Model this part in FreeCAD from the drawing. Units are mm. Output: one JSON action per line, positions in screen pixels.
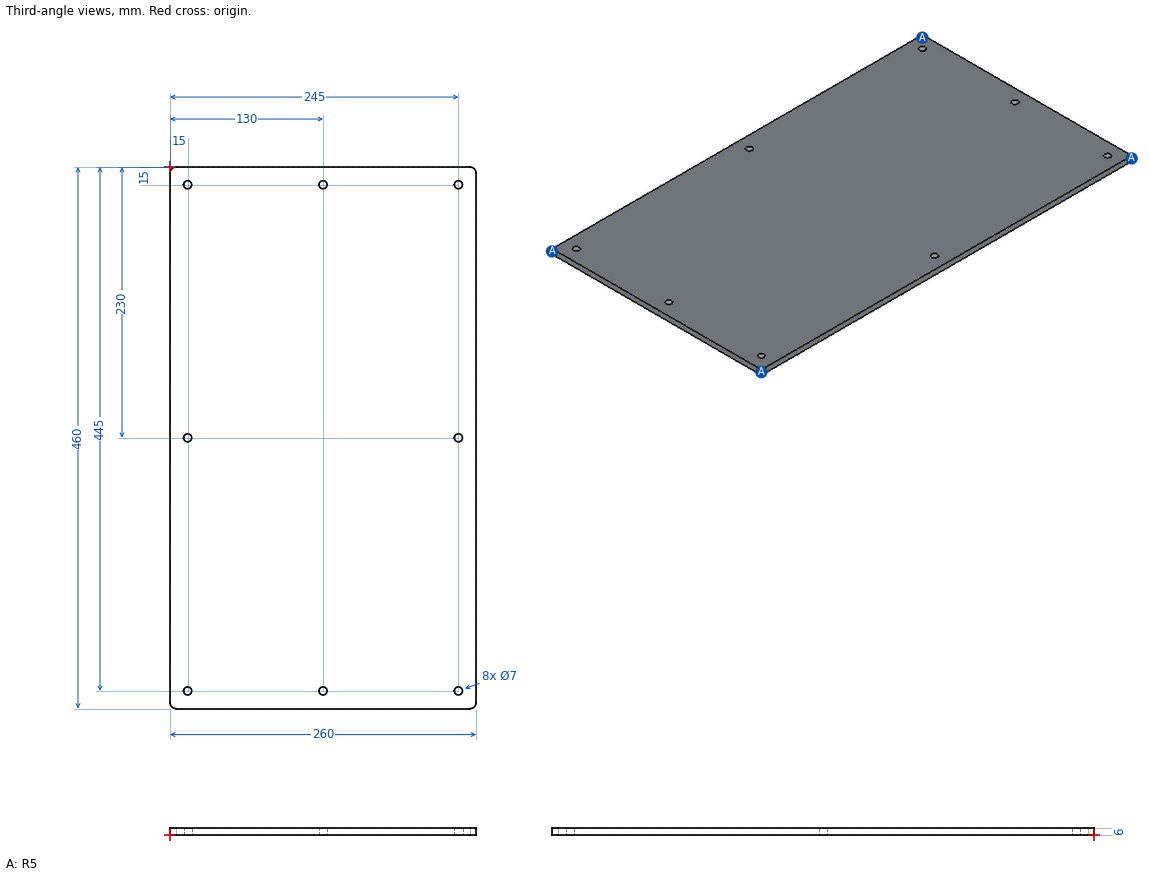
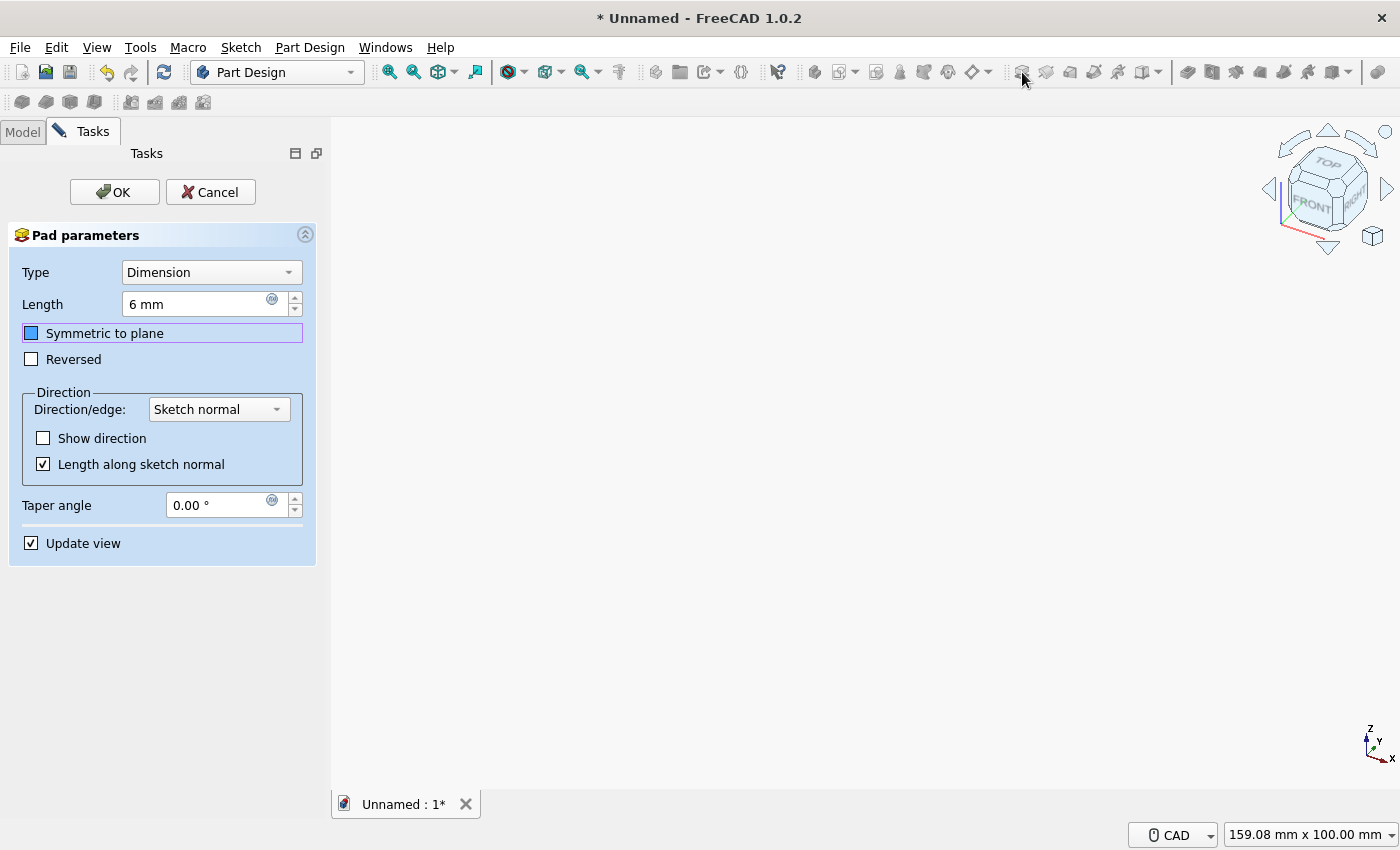
{"action": "left_click", "coordinate": [115, 192]}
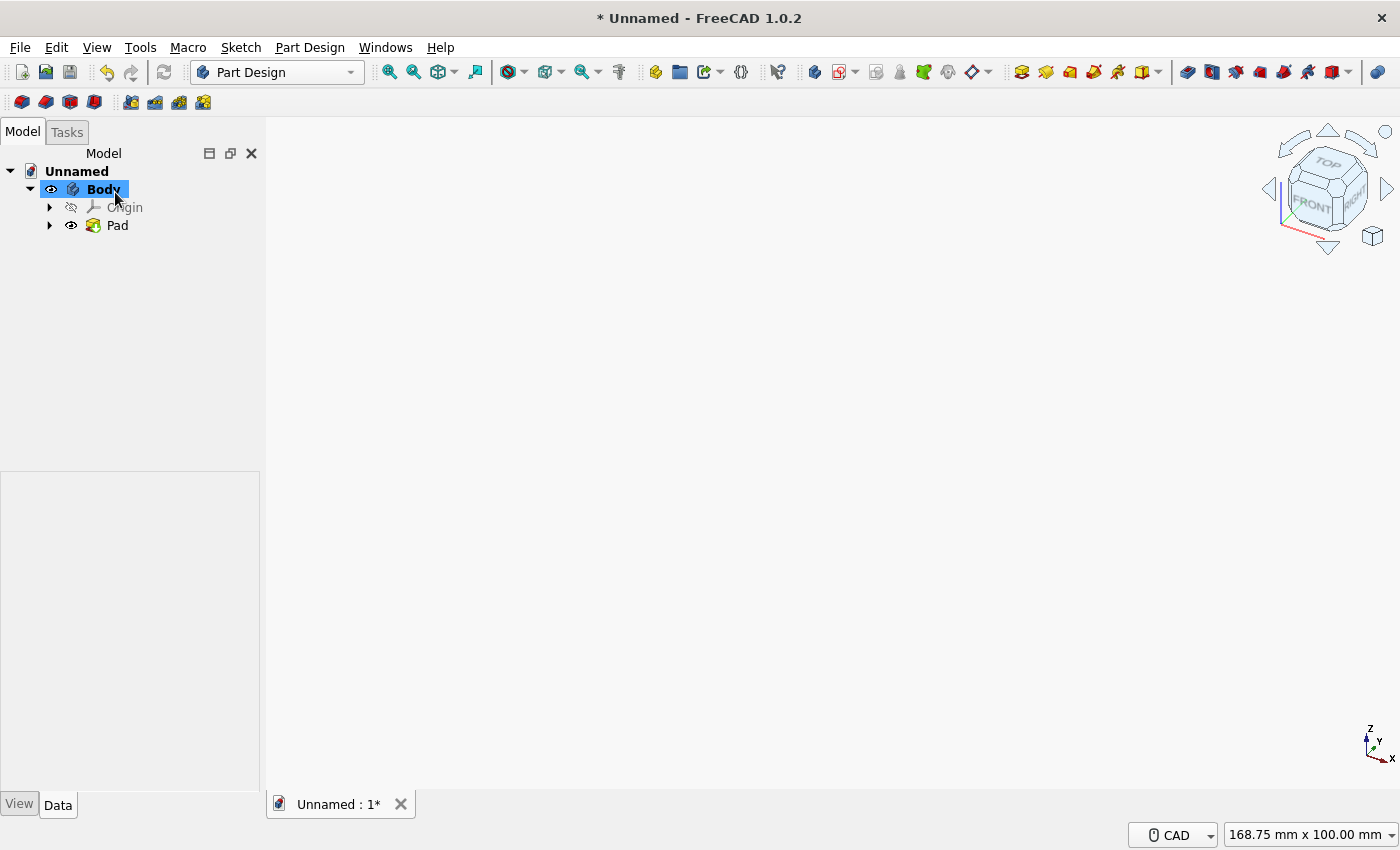
{"action": "key", "text": "v f"}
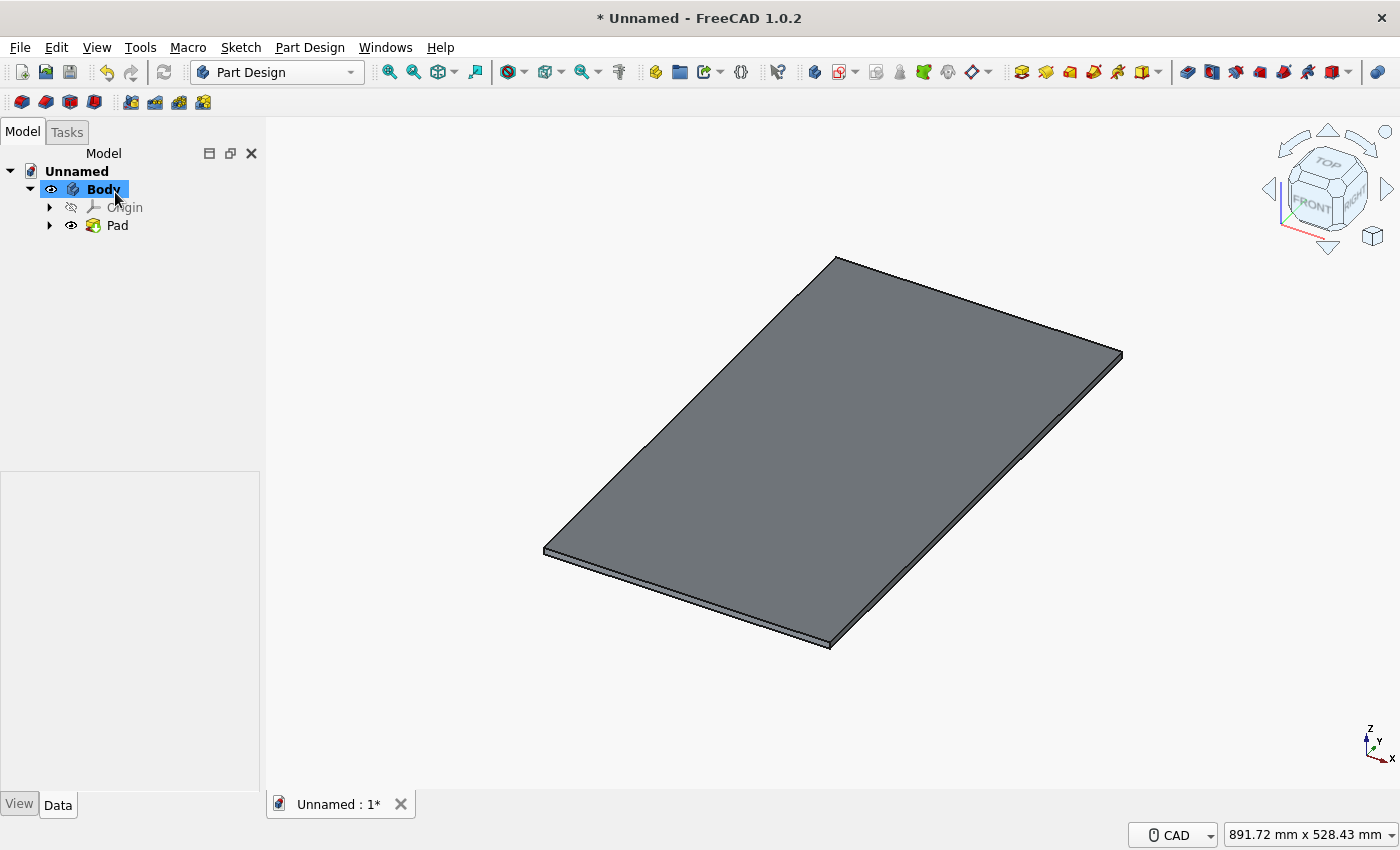
{"action": "scroll", "coordinate": [836, 259], "scroll_direction": "up", "scroll_amount": 9}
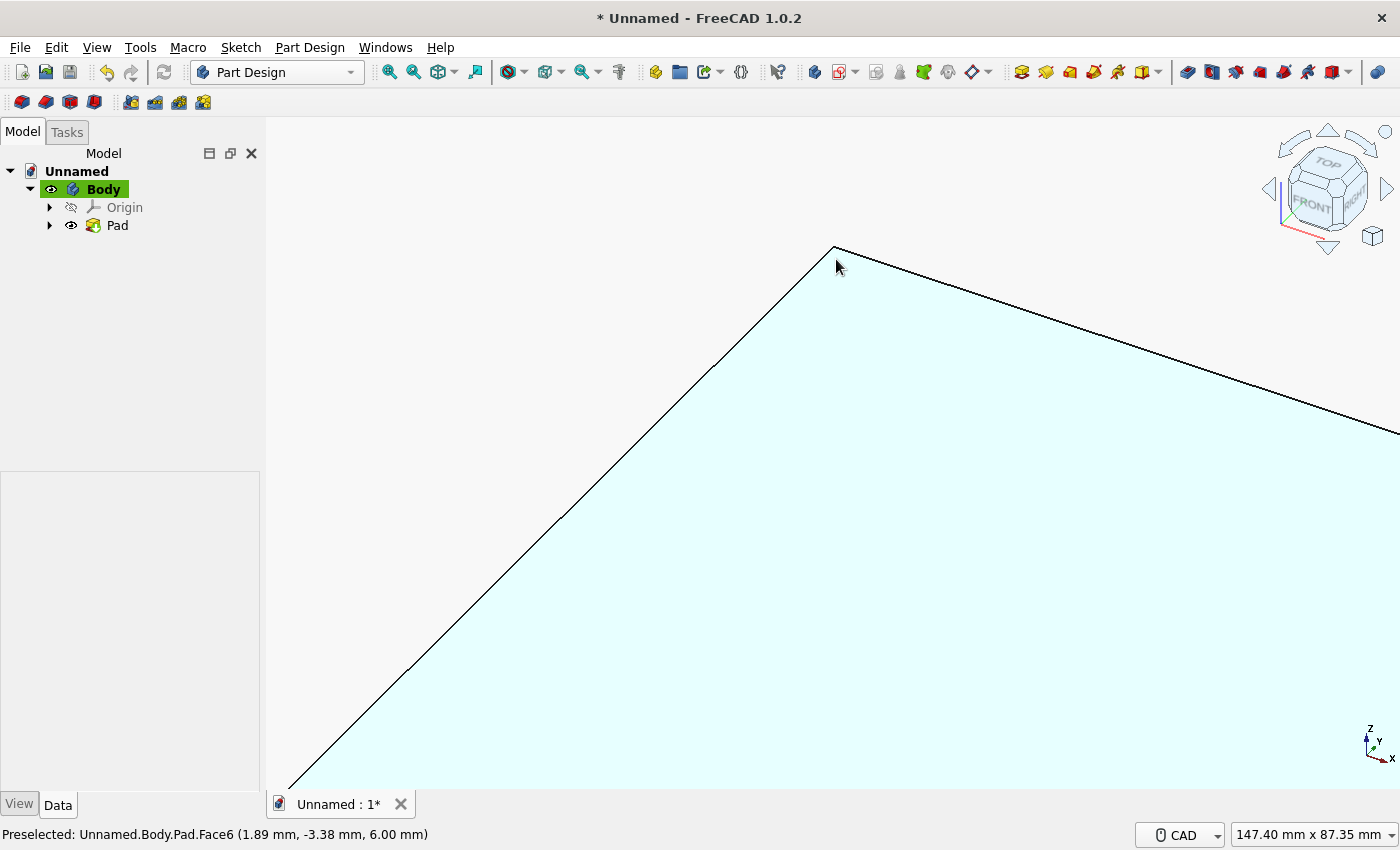
{"action": "key", "text": "v f"}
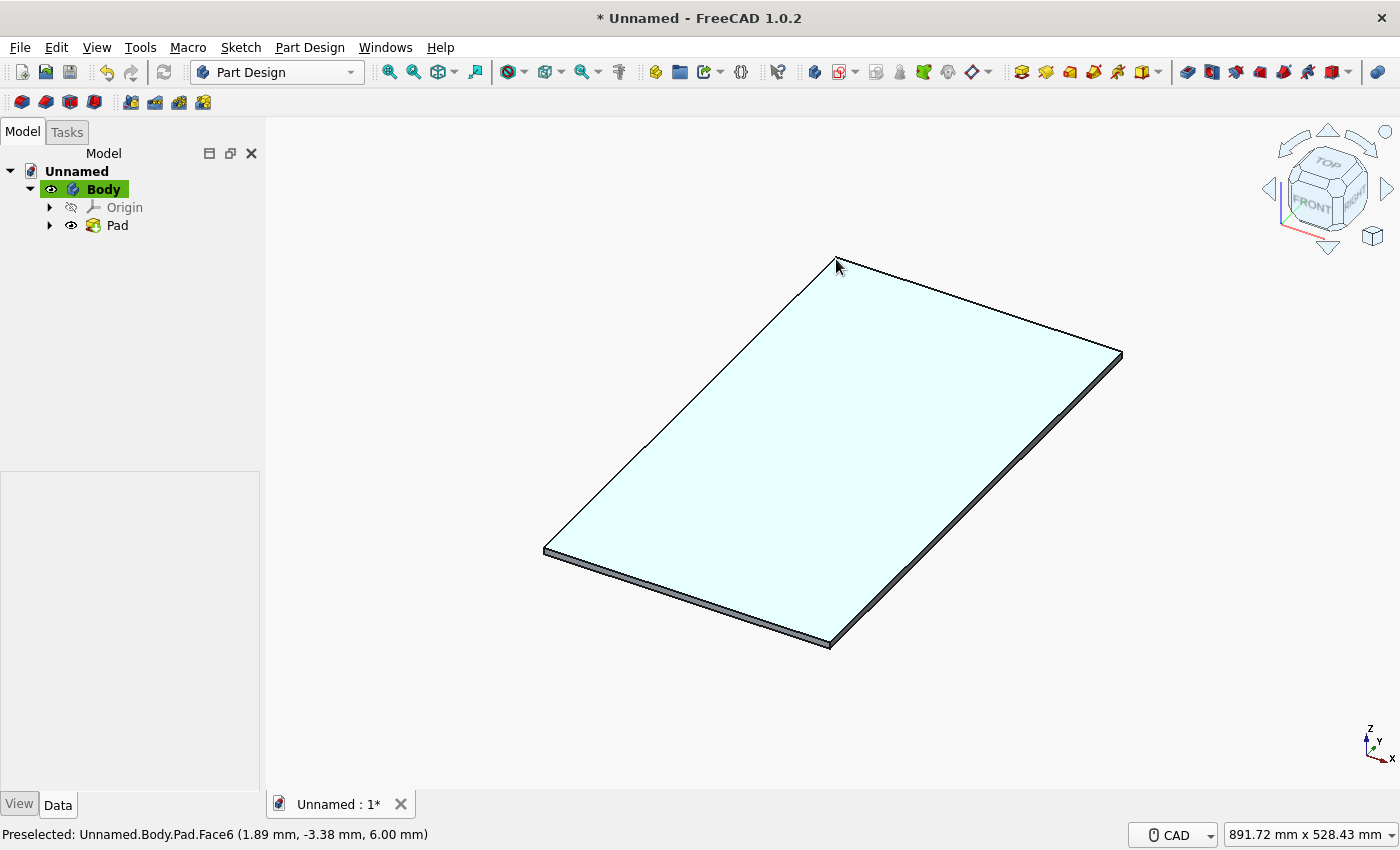
{"action": "key", "text": "0"}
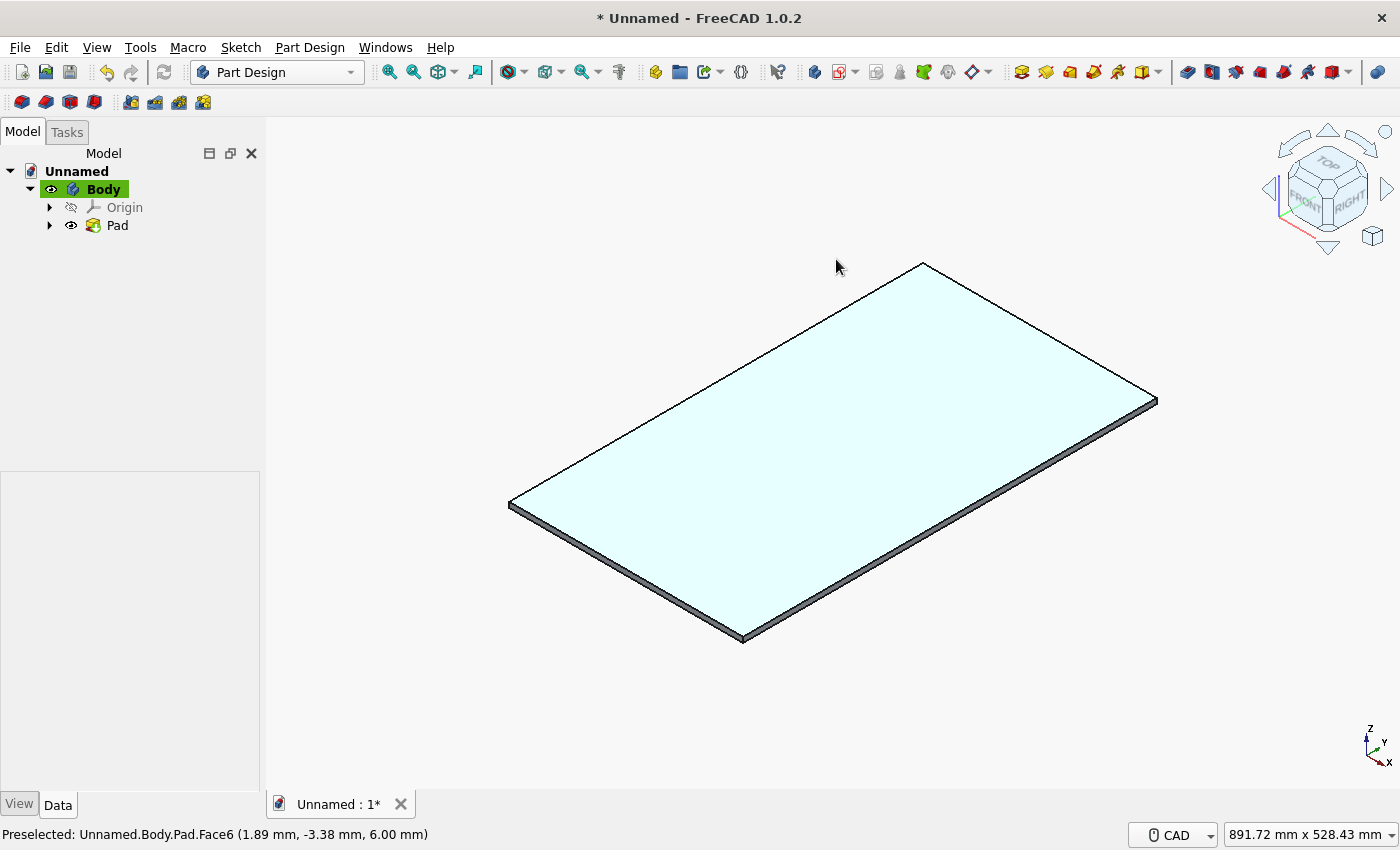
{"action": "scroll", "coordinate": [923, 265], "scroll_direction": "up", "scroll_amount": 9}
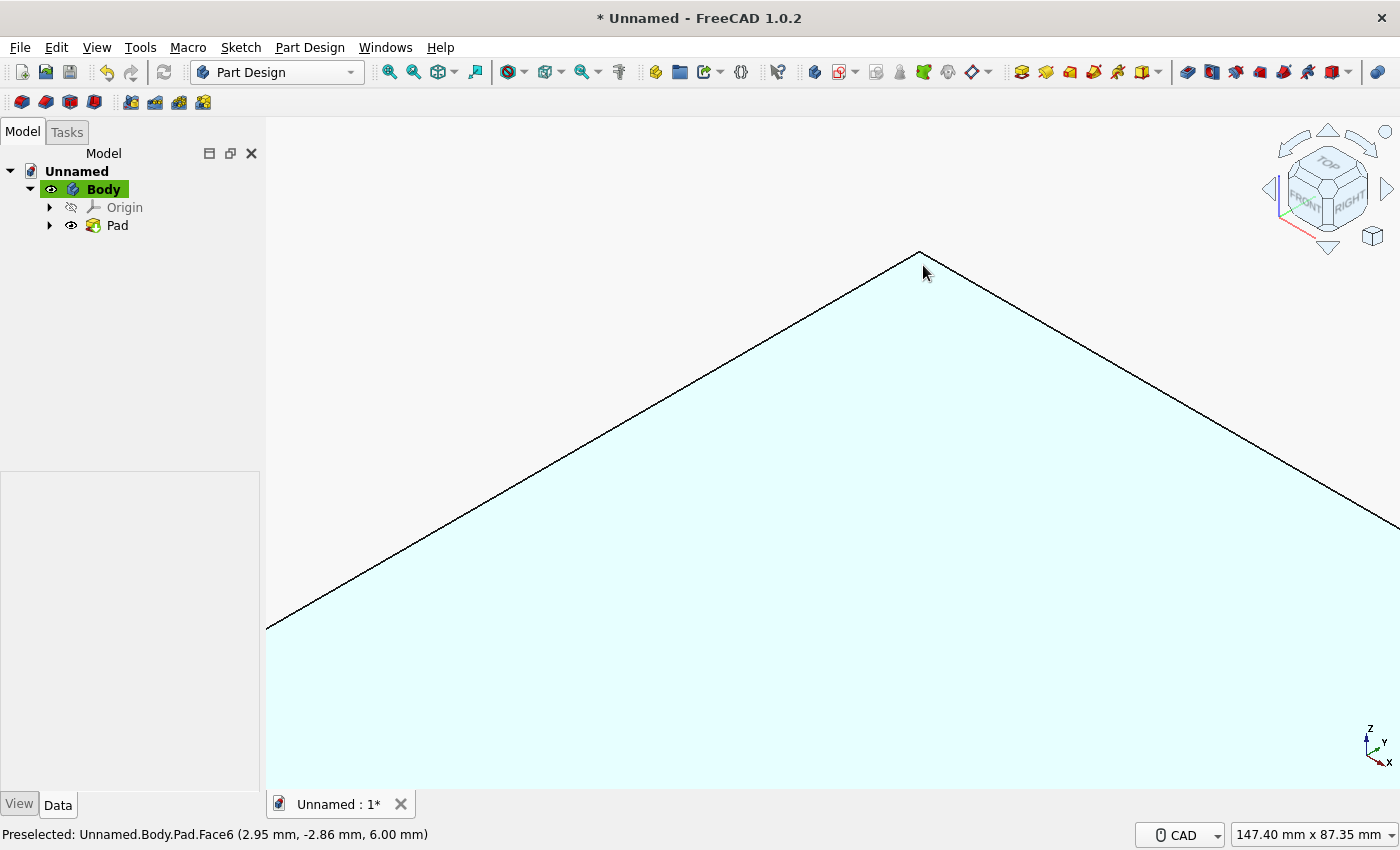
{"action": "key", "text": "v f"}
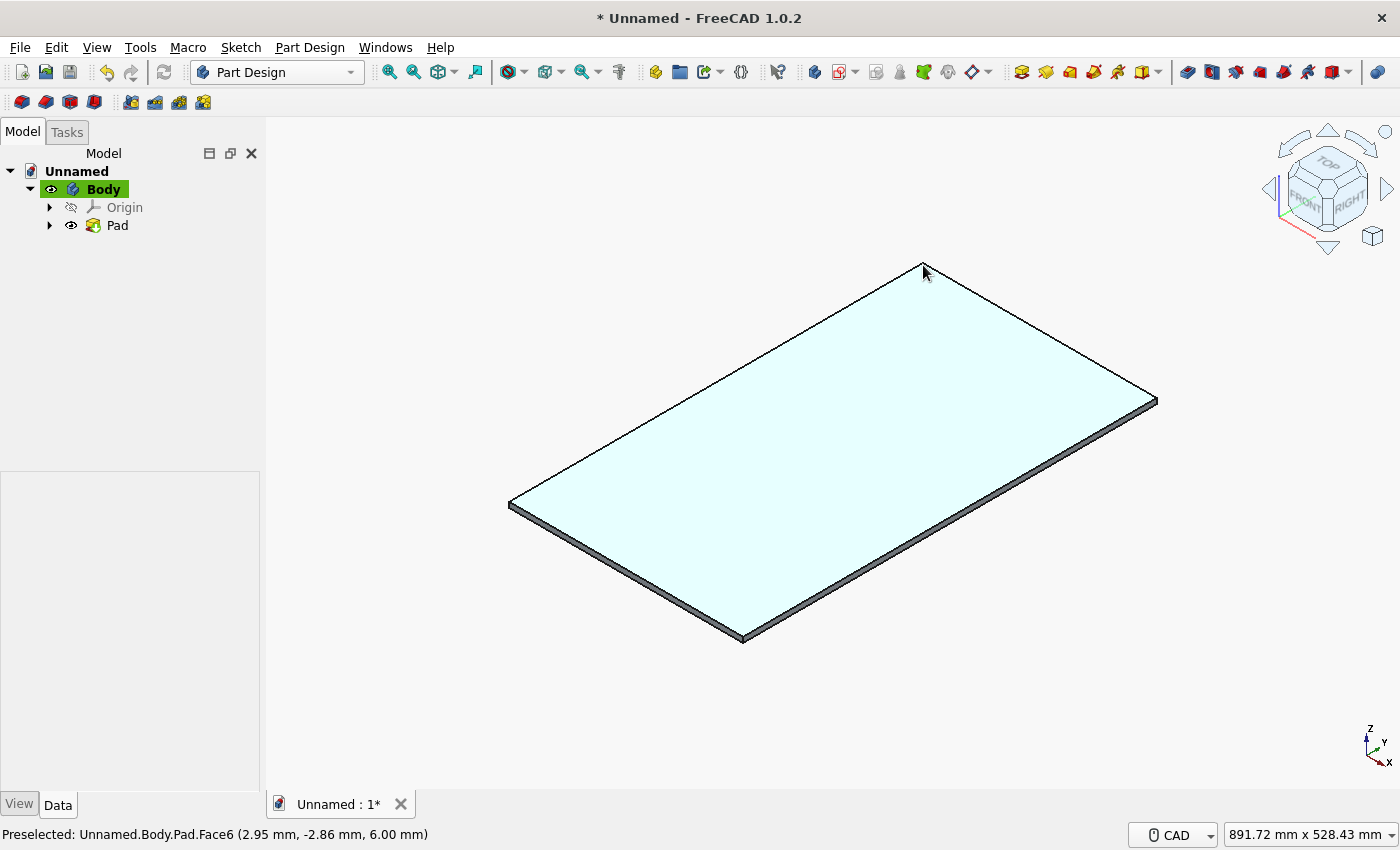
{"action": "key", "text": "2"}